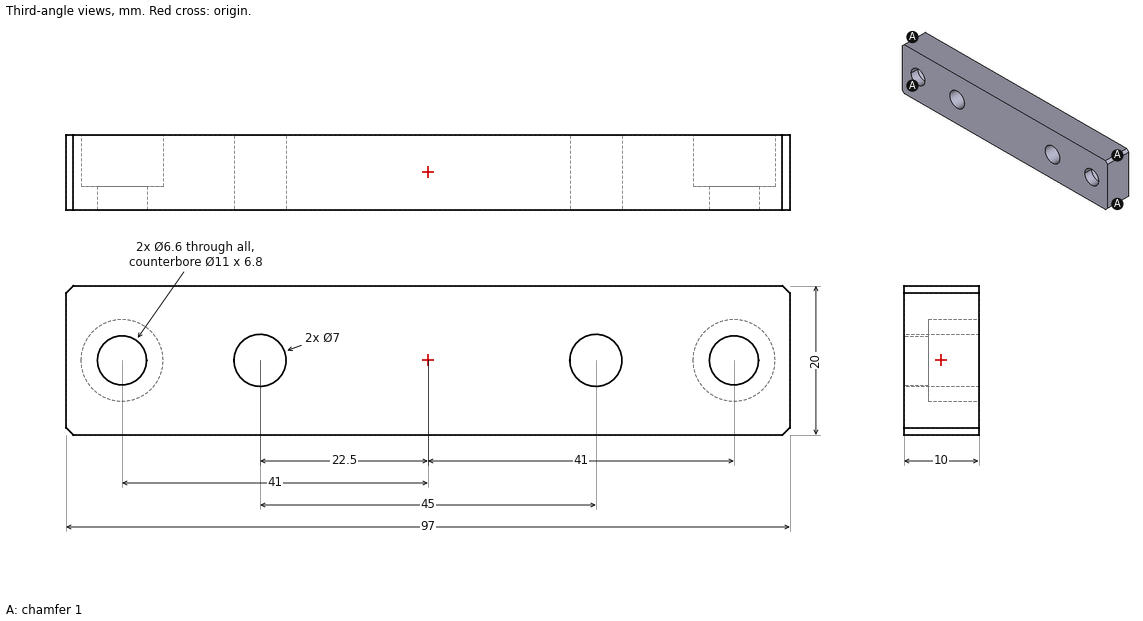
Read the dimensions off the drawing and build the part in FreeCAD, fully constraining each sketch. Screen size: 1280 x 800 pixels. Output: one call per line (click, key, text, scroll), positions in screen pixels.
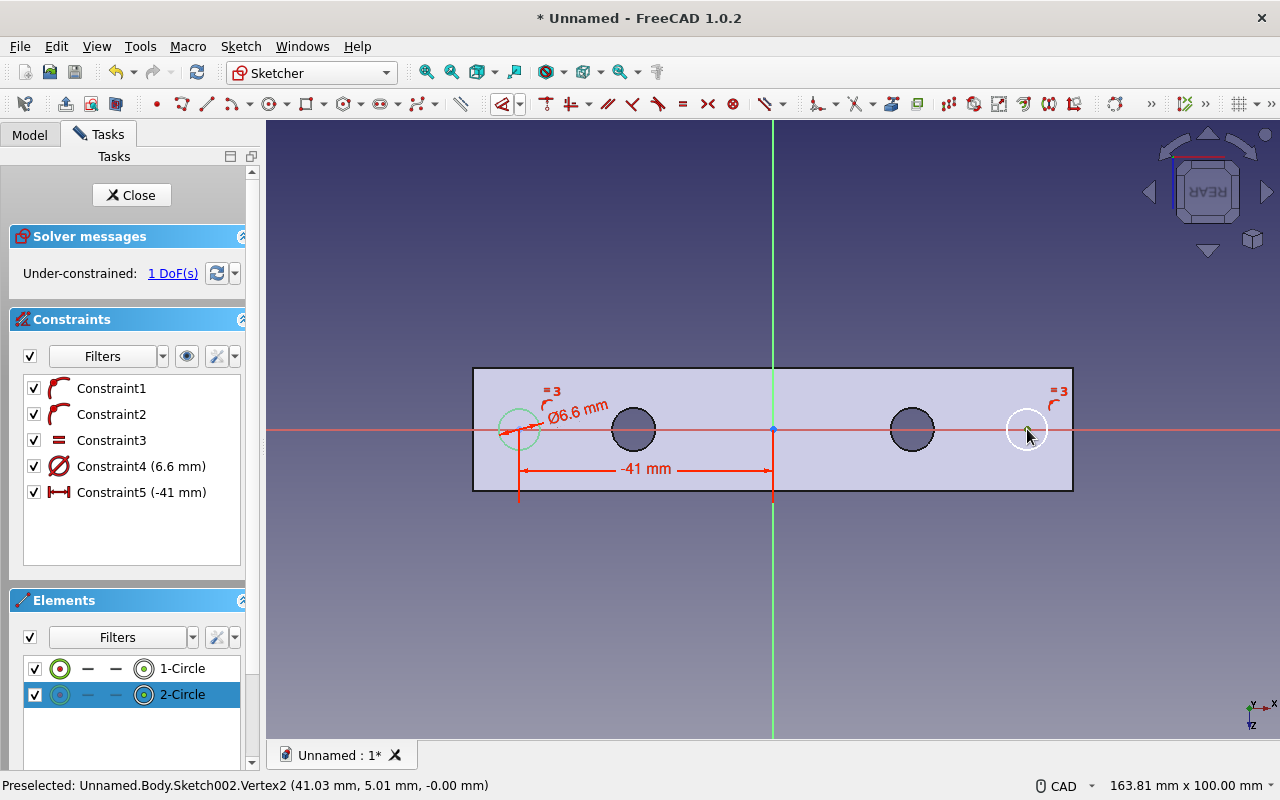
click(520, 104)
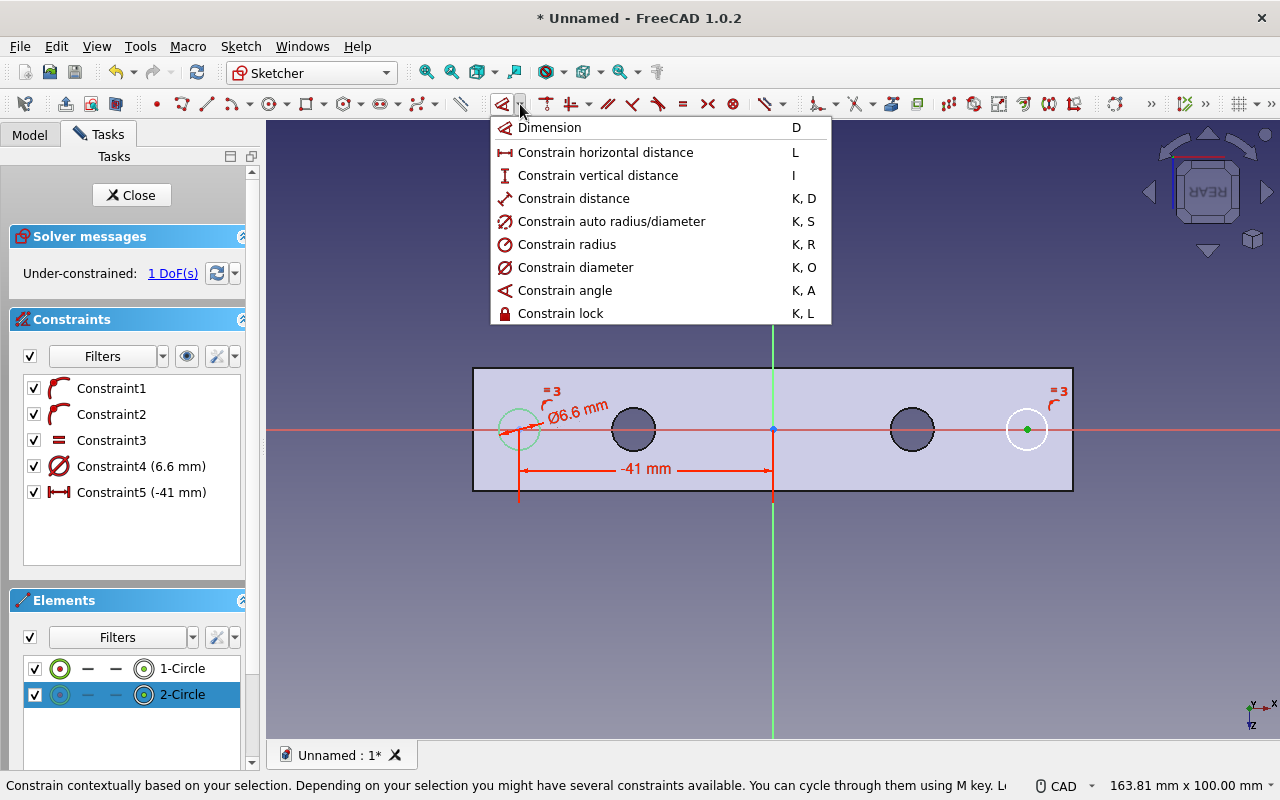
click(661, 152)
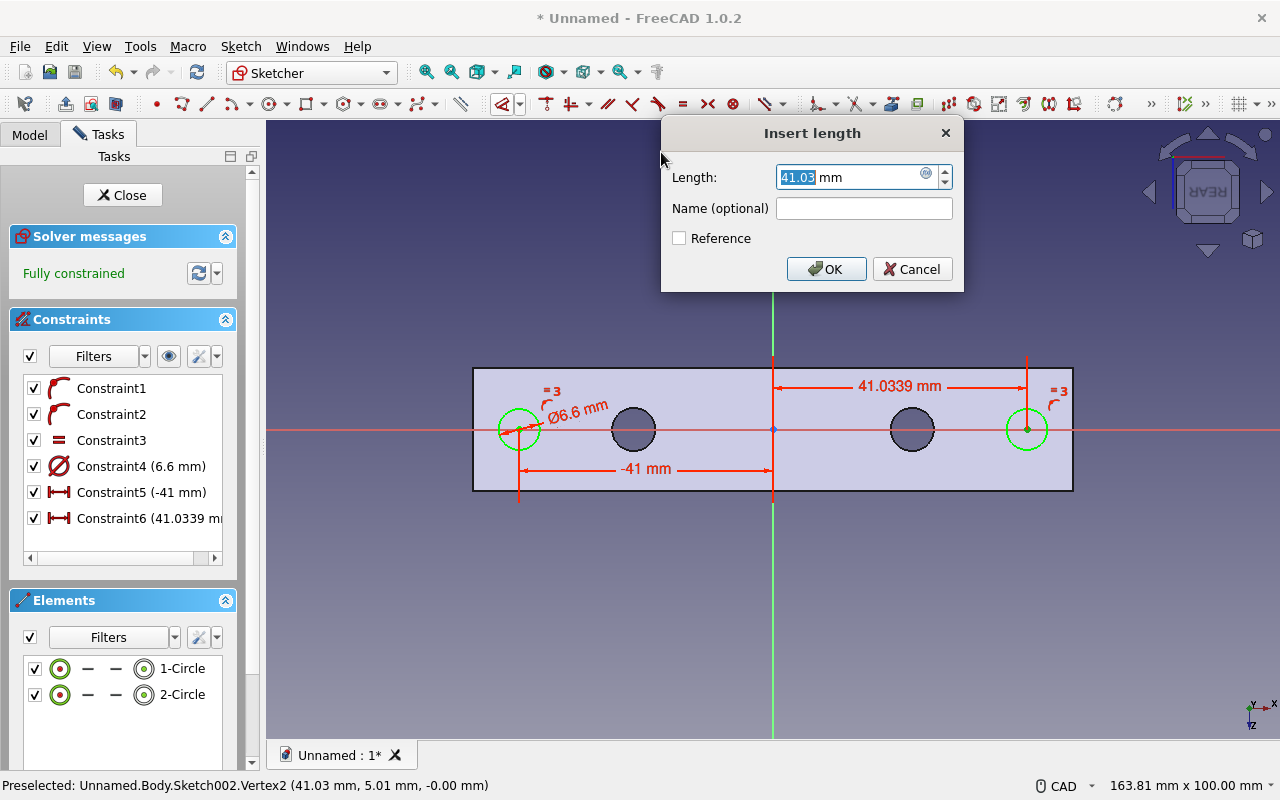
text(41)
key(Return)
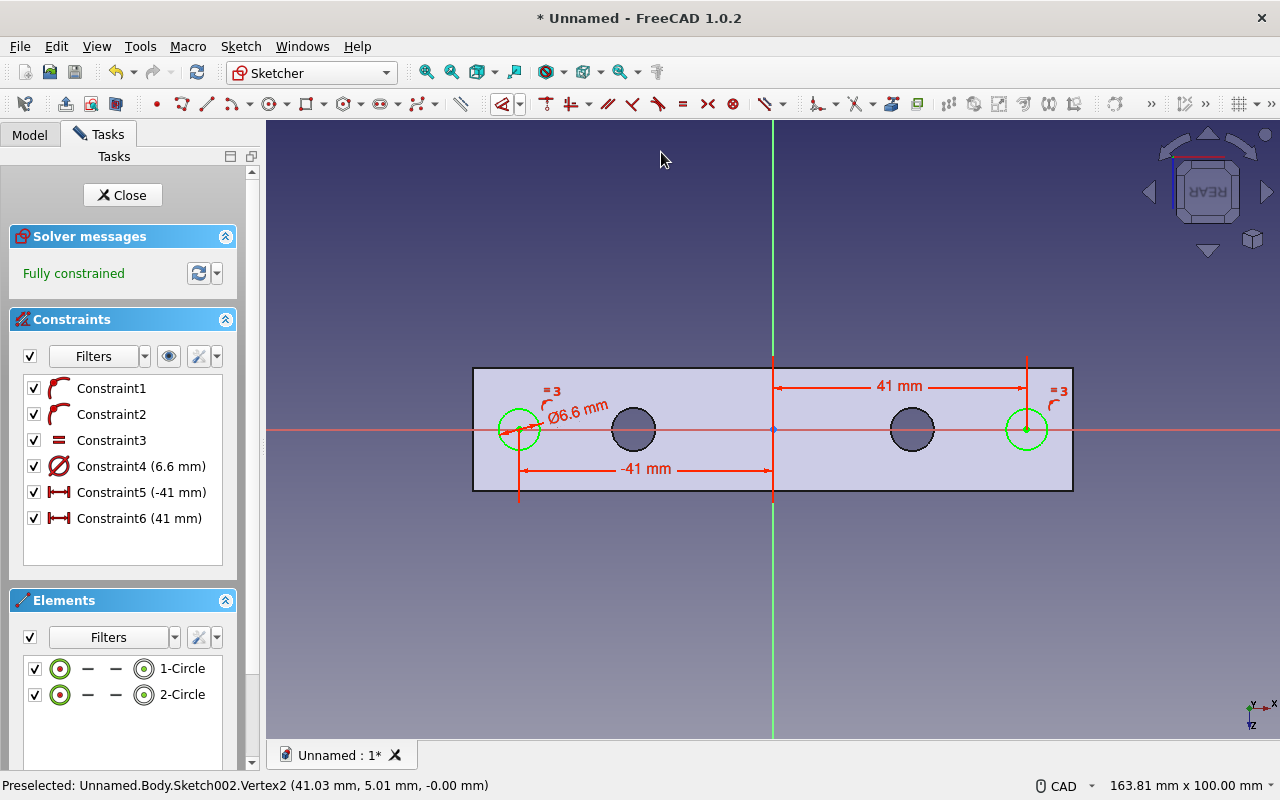
click(123, 195)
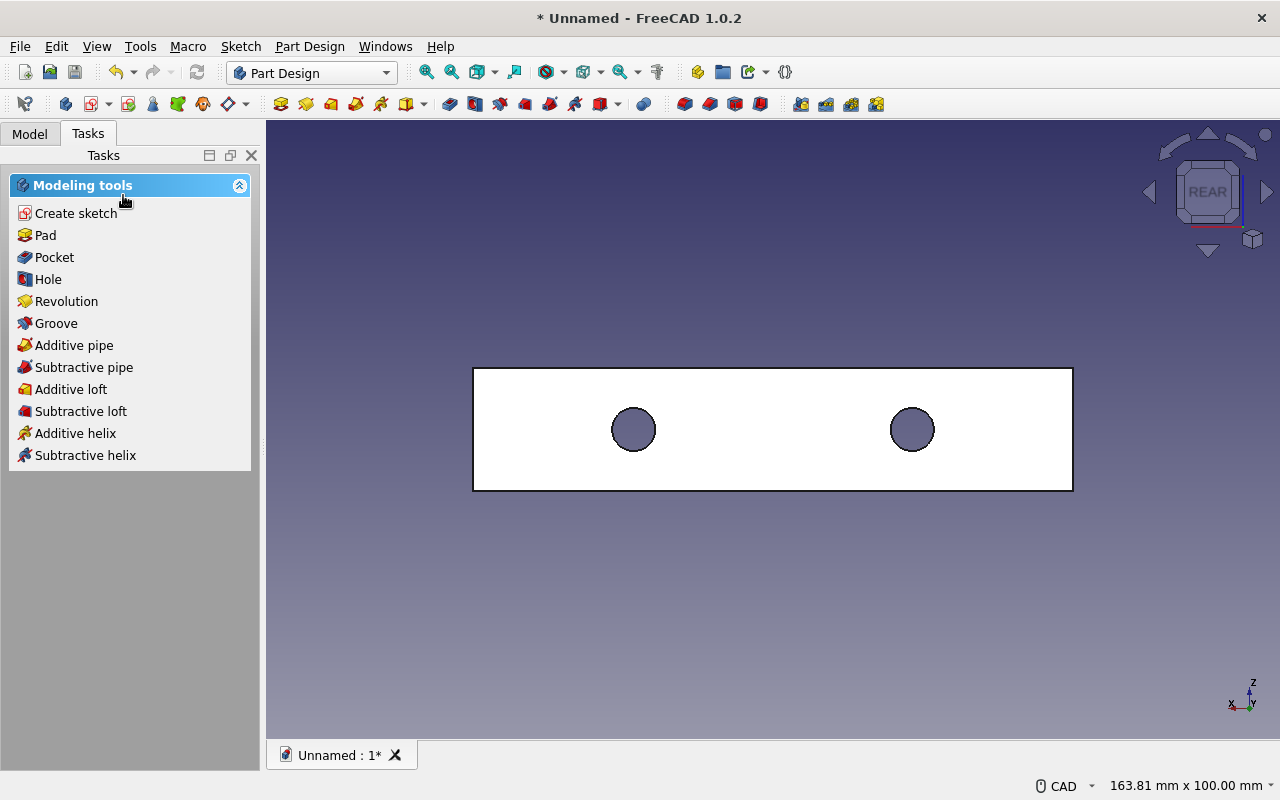
click(475, 104)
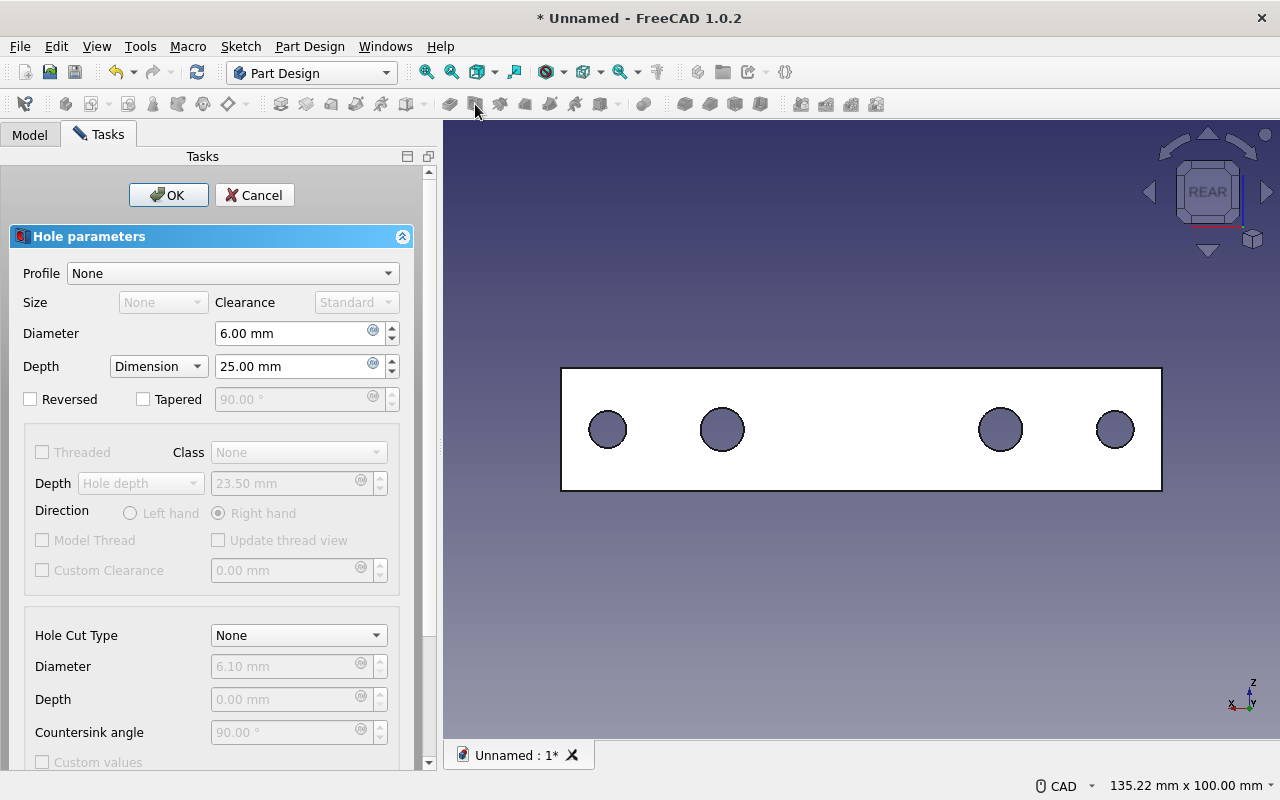
triple_click(300, 334)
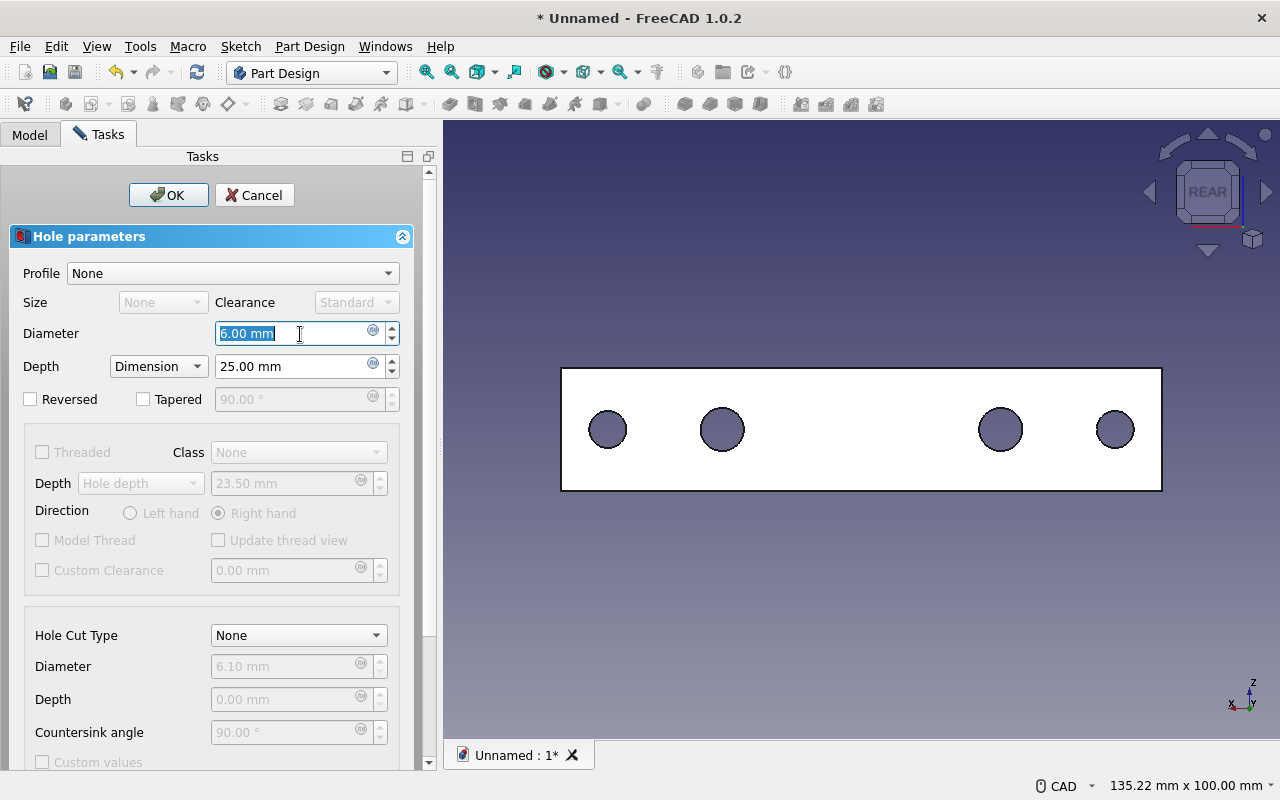
text(6.6)
key(Tab)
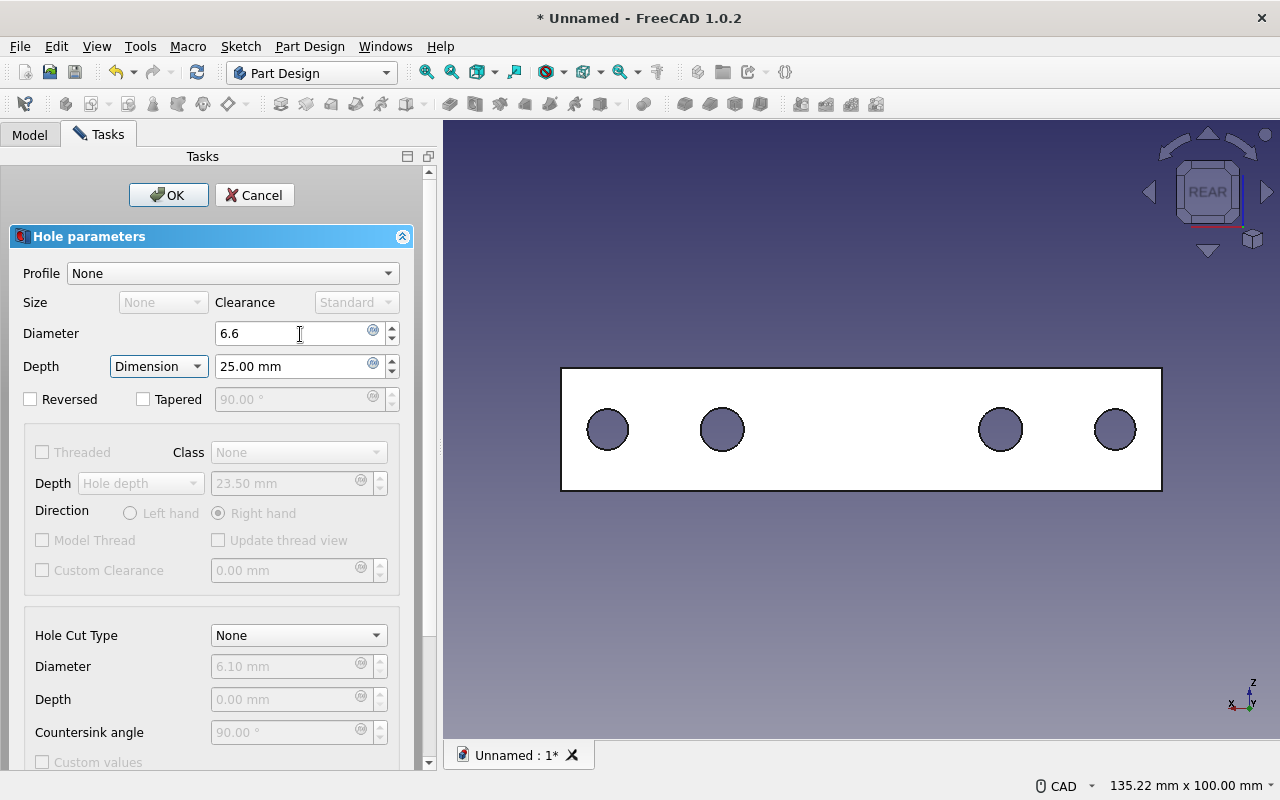
click(160, 366)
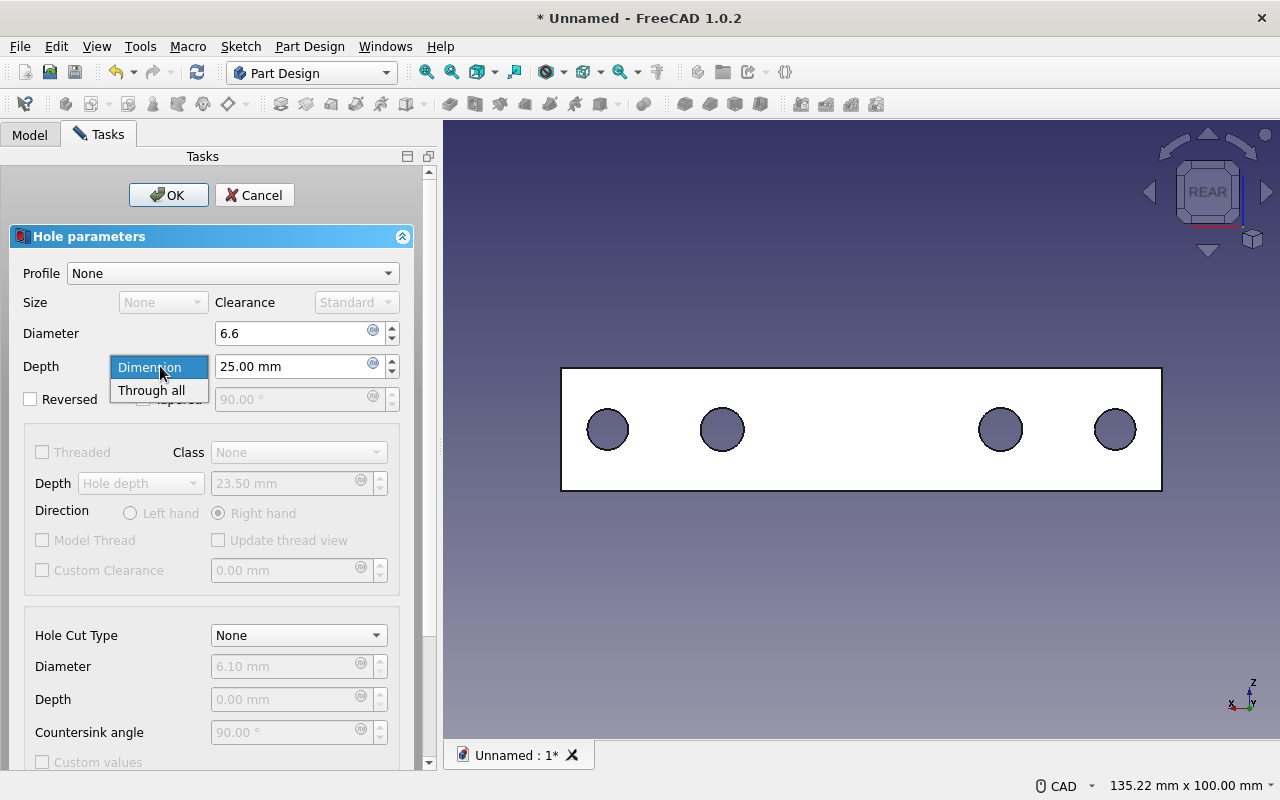
click(158, 390)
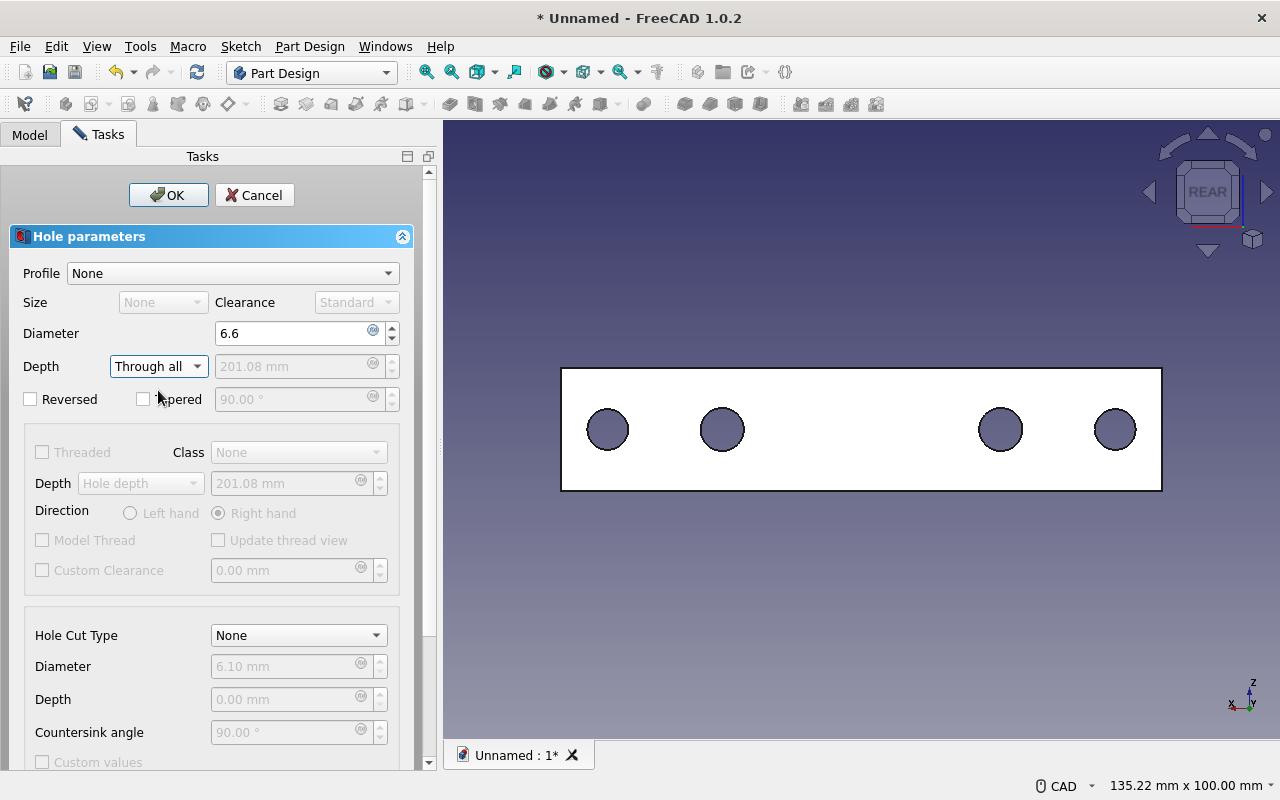
click(300, 636)